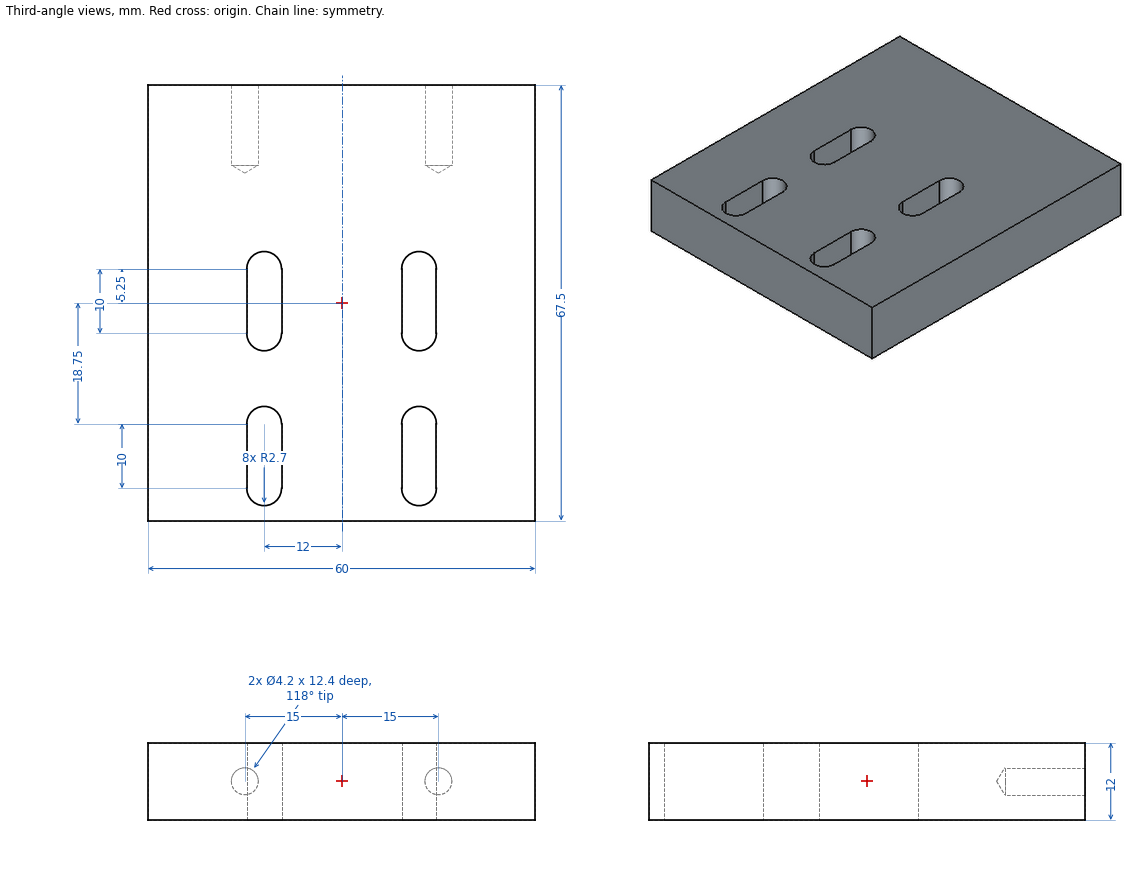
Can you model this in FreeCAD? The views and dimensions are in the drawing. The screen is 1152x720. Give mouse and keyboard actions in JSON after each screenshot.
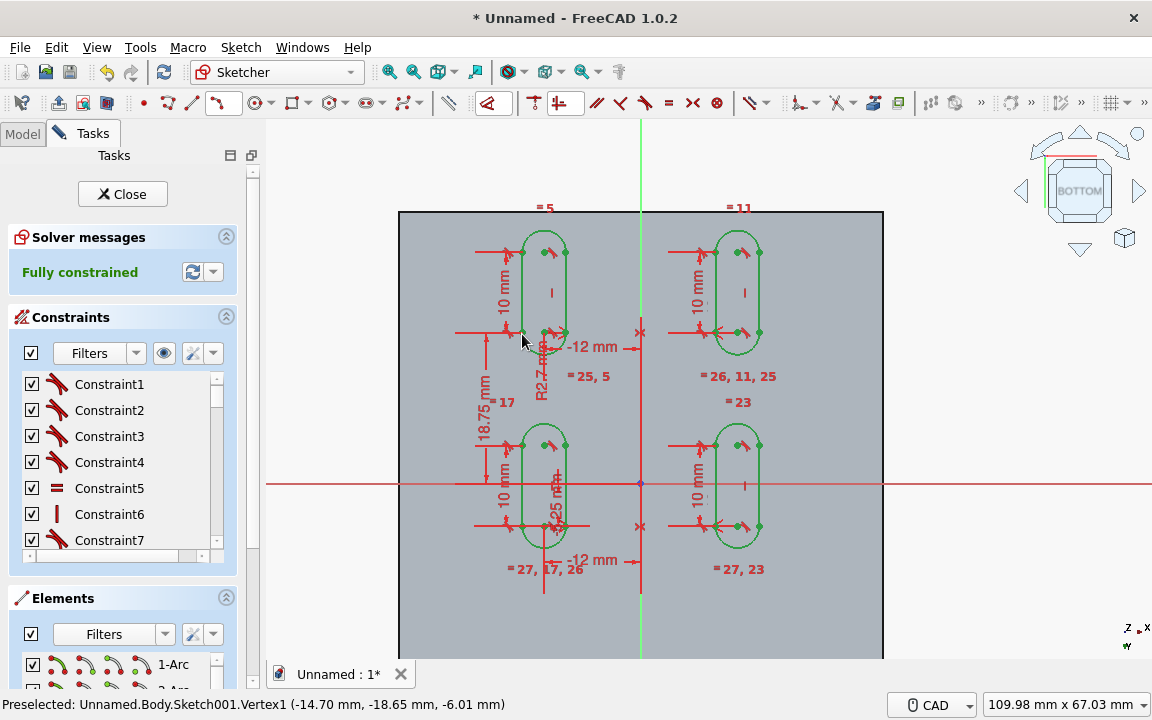
{"action": "left_click", "coordinate": [123, 194]}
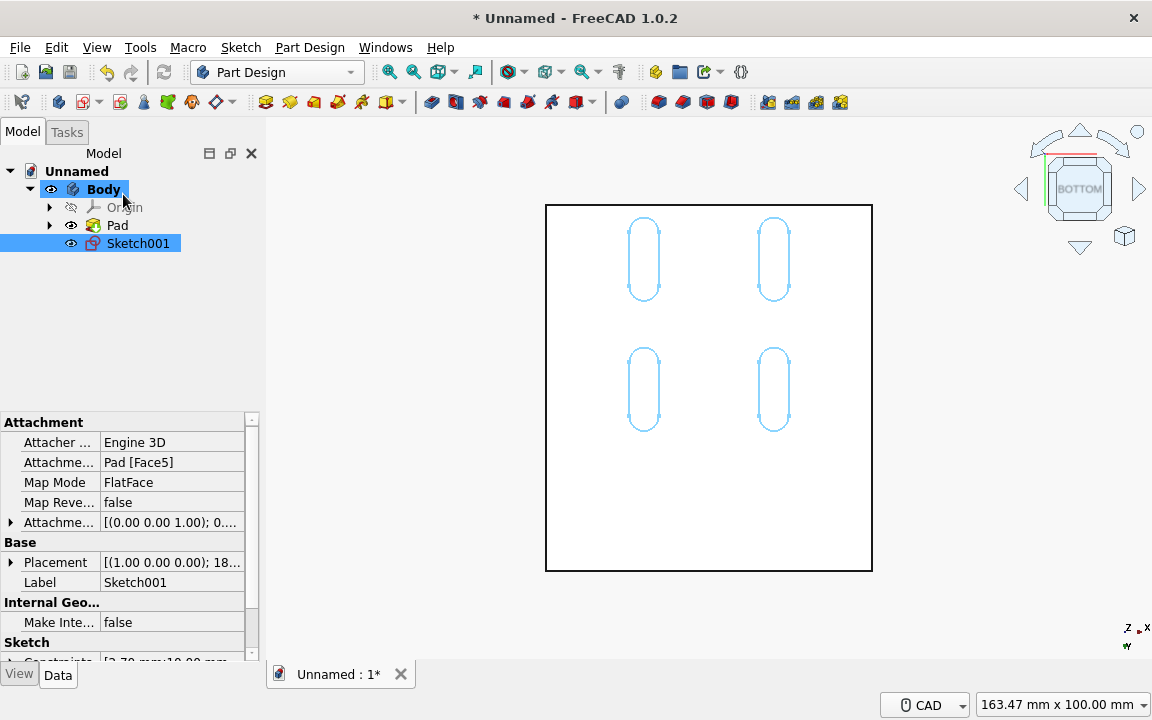
{"action": "left_click", "coordinate": [432, 102]}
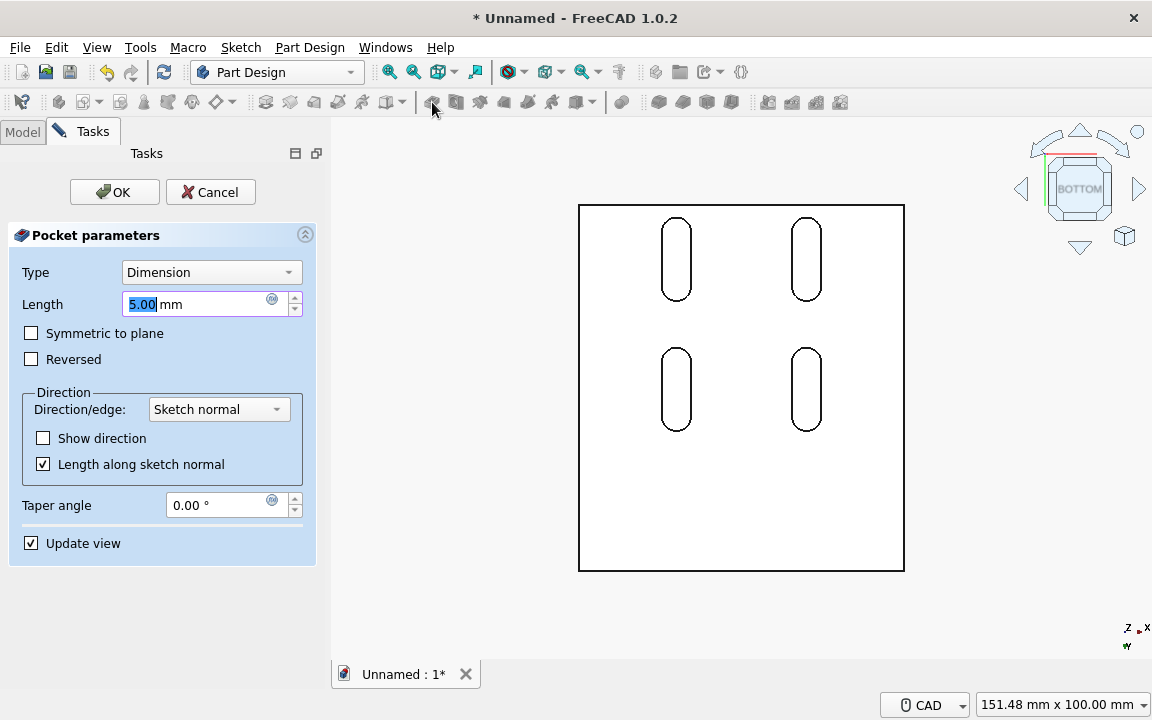
{"action": "left_click", "coordinate": [212, 272]}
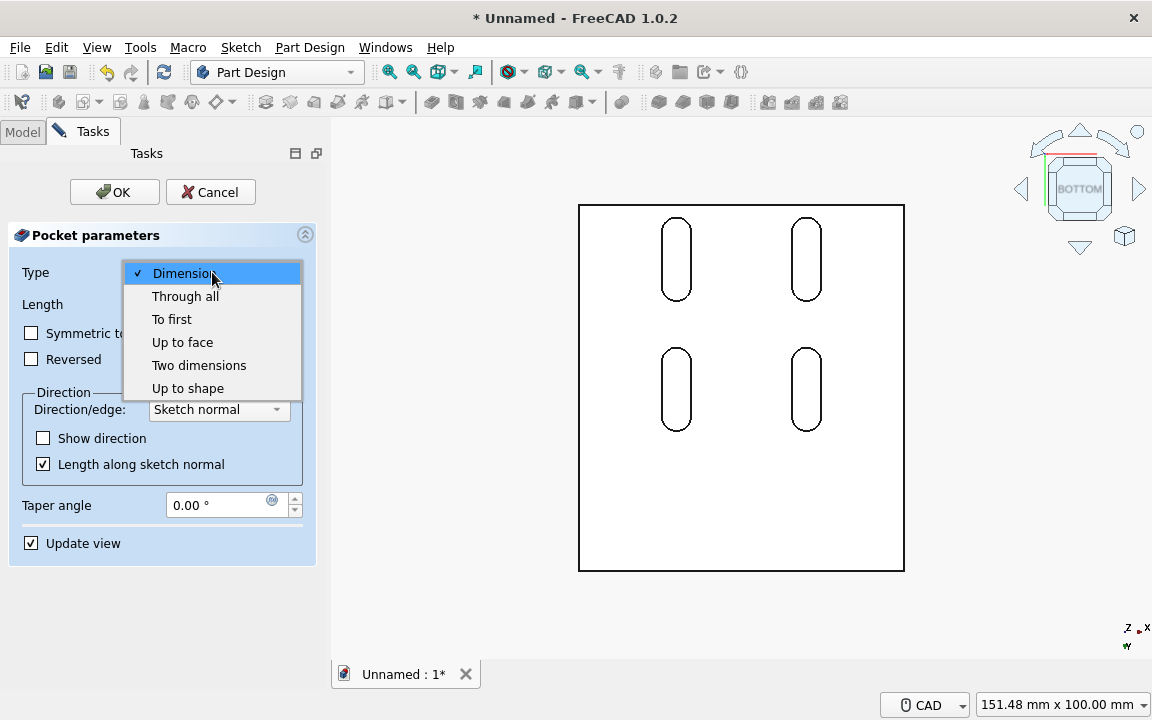
{"action": "left_click", "coordinate": [212, 296]}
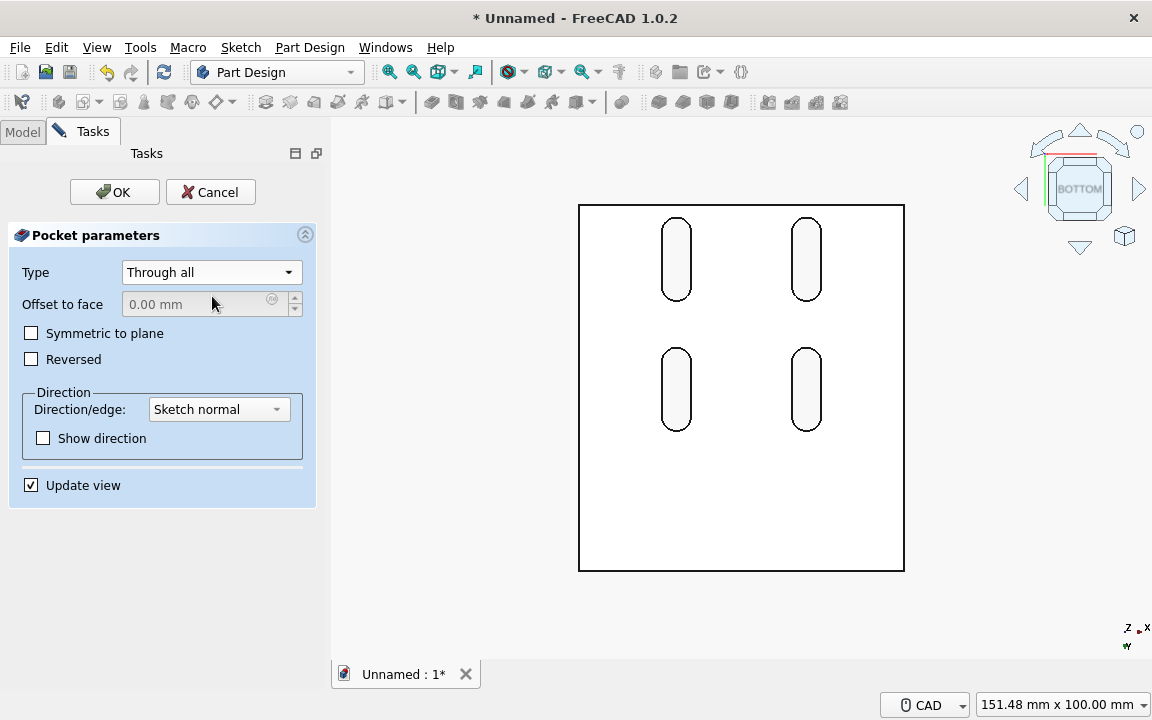
{"action": "left_click", "coordinate": [115, 192]}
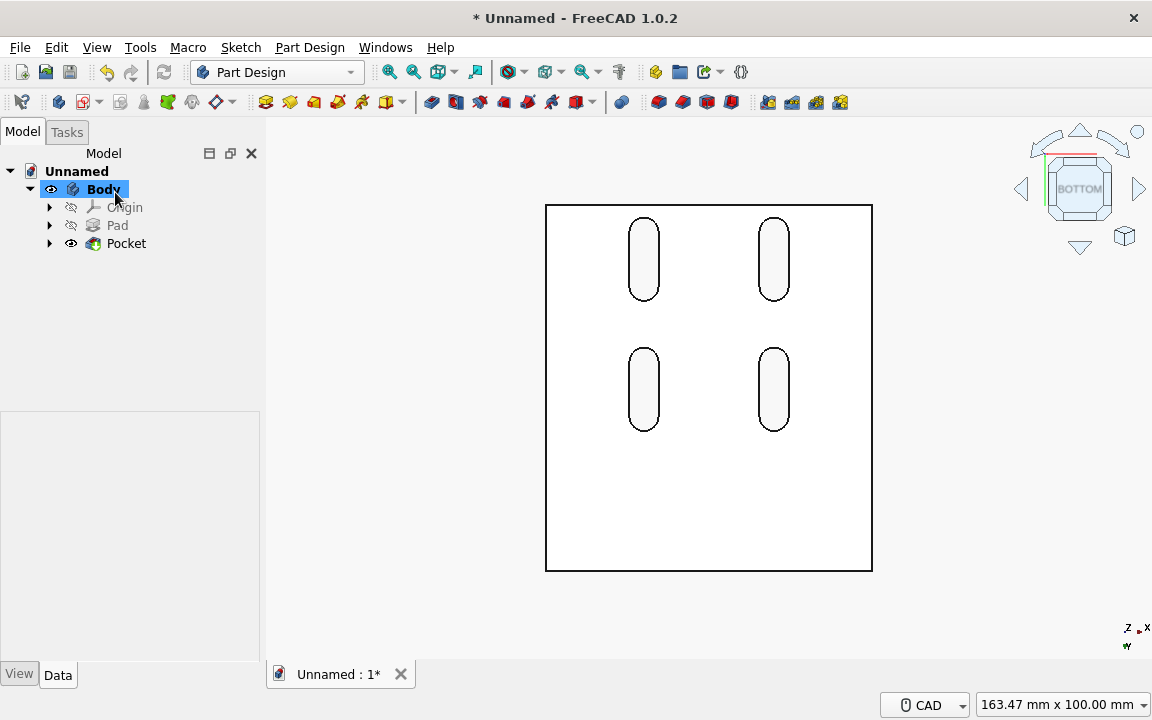
{"action": "key", "text": "4"}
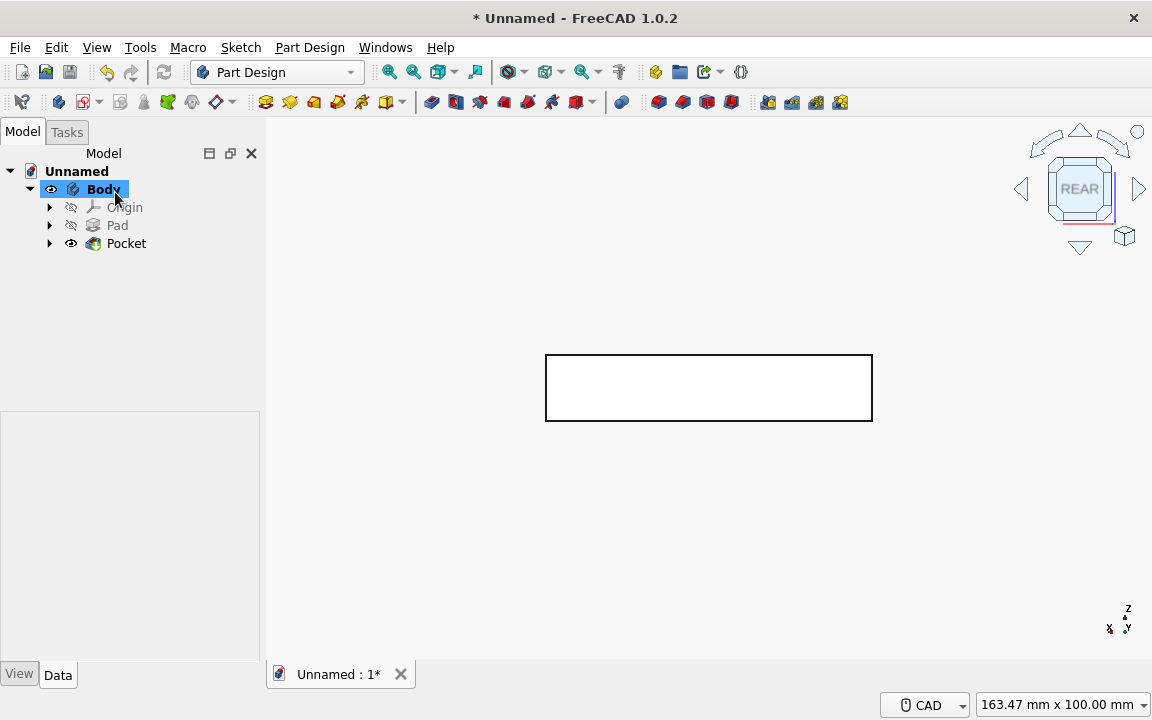
{"action": "key", "text": "v f"}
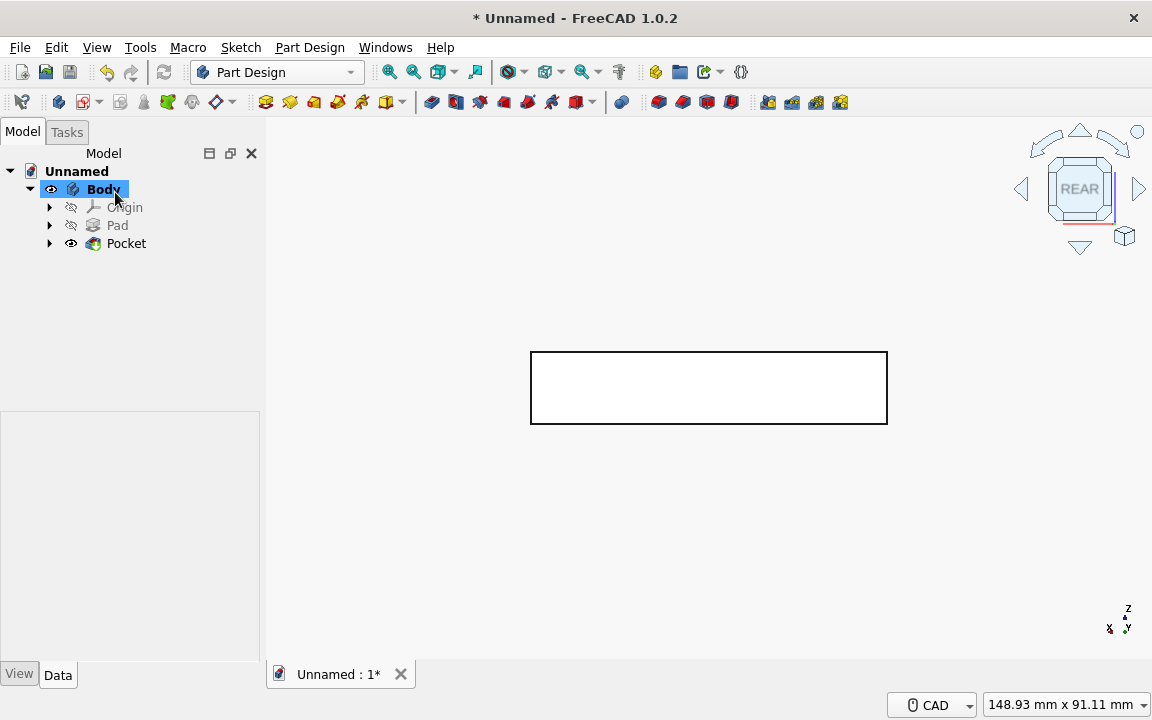
{"action": "left_click", "coordinate": [607, 387]}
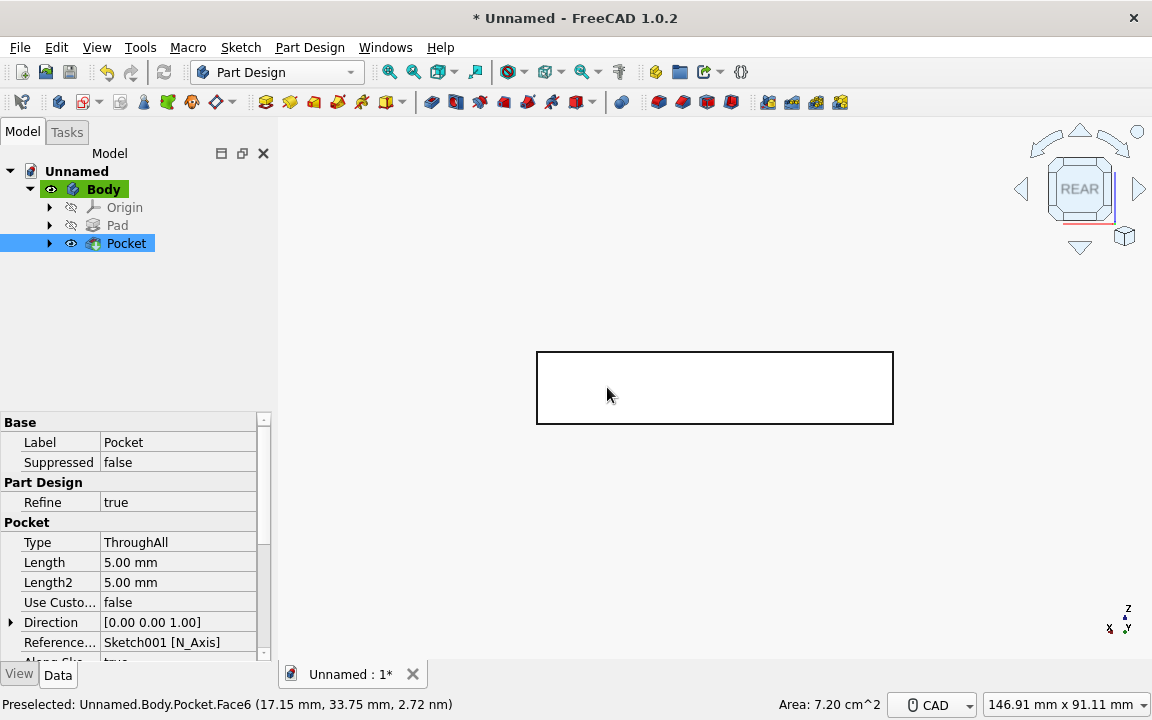
{"action": "left_click", "coordinate": [84, 102]}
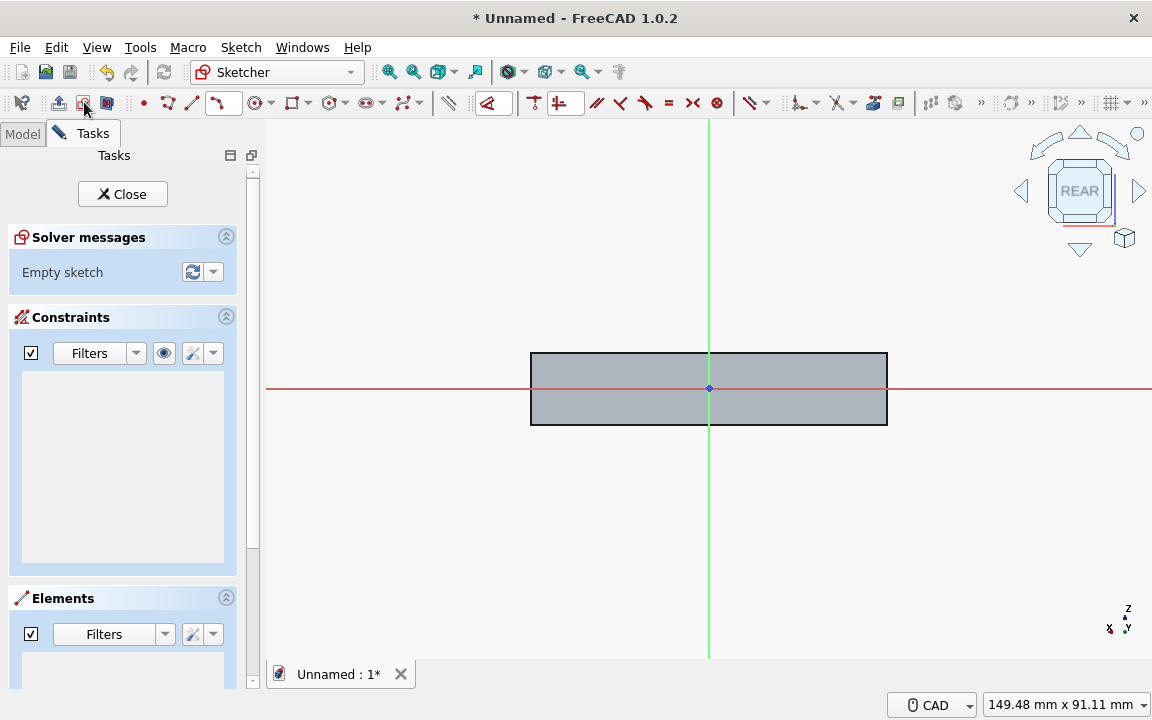
{"action": "scroll", "coordinate": [765, 389], "scroll_direction": "up", "scroll_amount": 4}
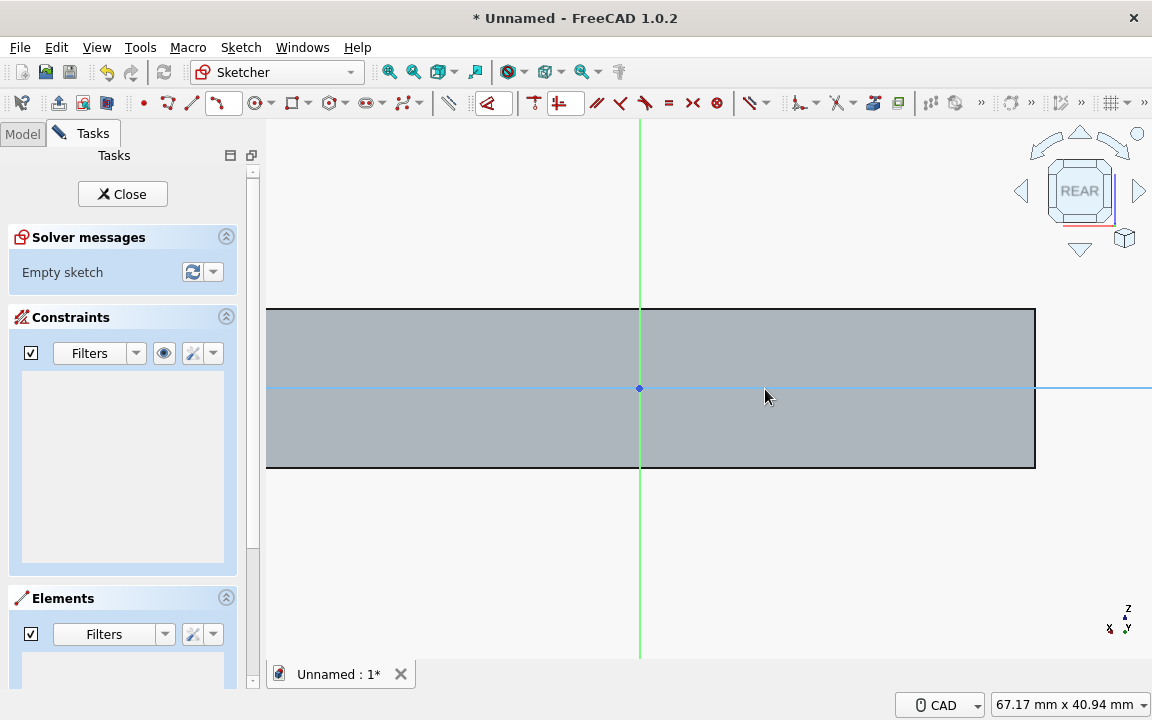
{"action": "left_click", "coordinate": [256, 104]}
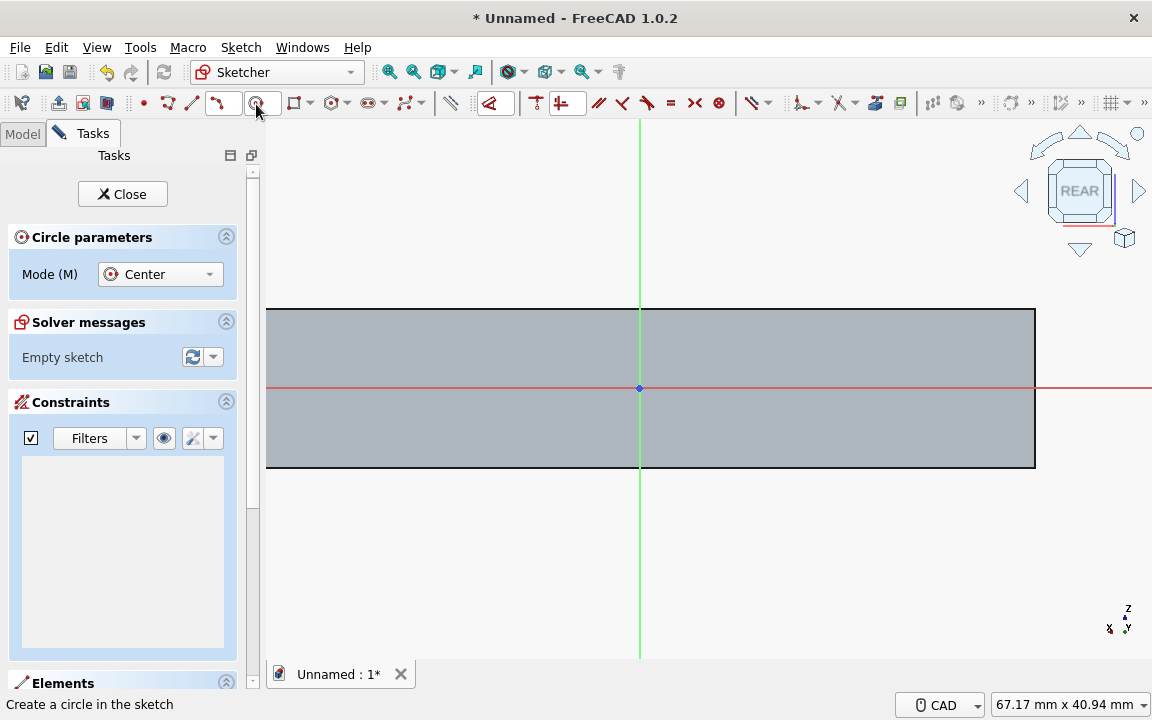
{"action": "left_click", "coordinate": [838, 388]}
{"action": "mouse_move", "coordinate": [857, 369]}